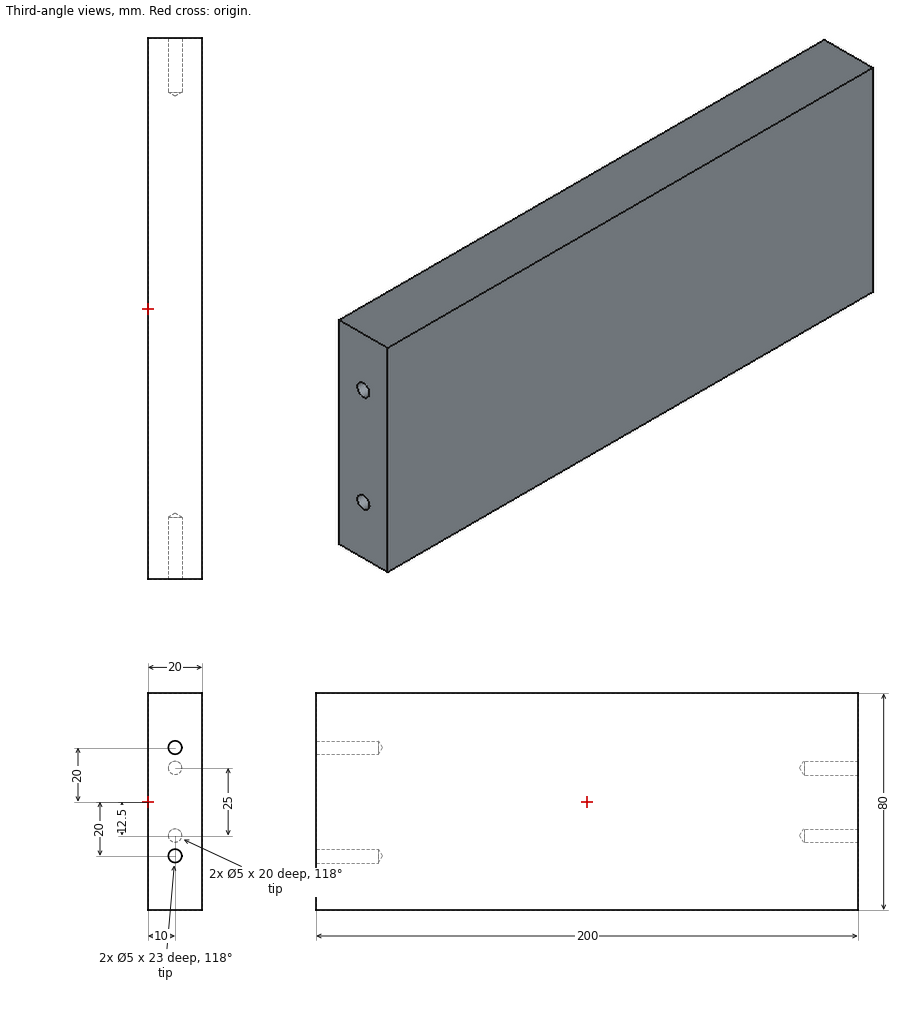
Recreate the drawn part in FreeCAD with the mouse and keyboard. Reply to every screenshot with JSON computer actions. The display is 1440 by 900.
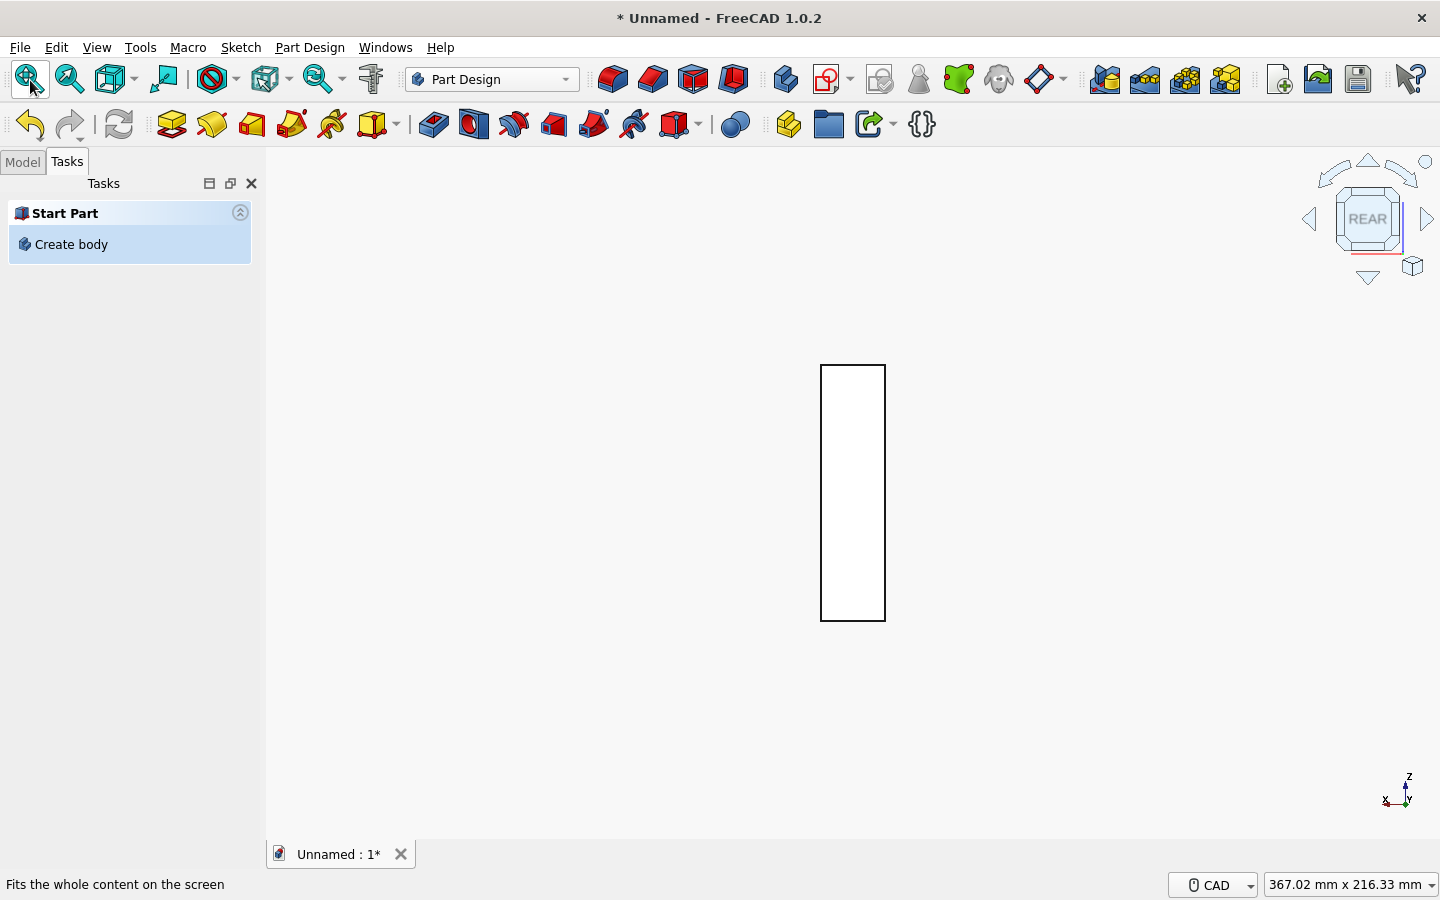
{"action": "left_click", "coordinate": [30, 80]}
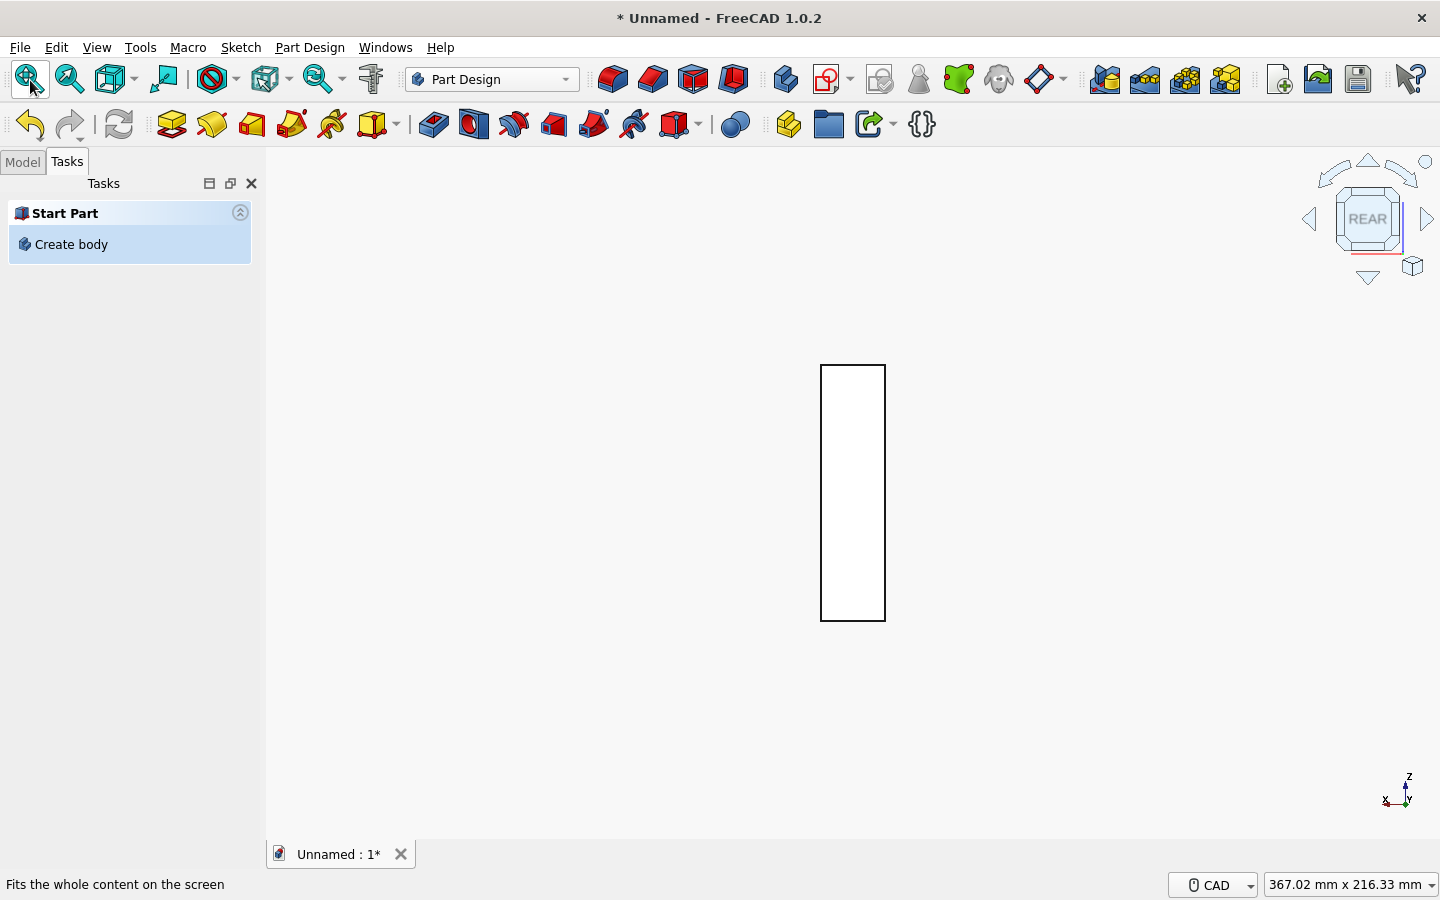
{"action": "left_click", "coordinate": [853, 565]}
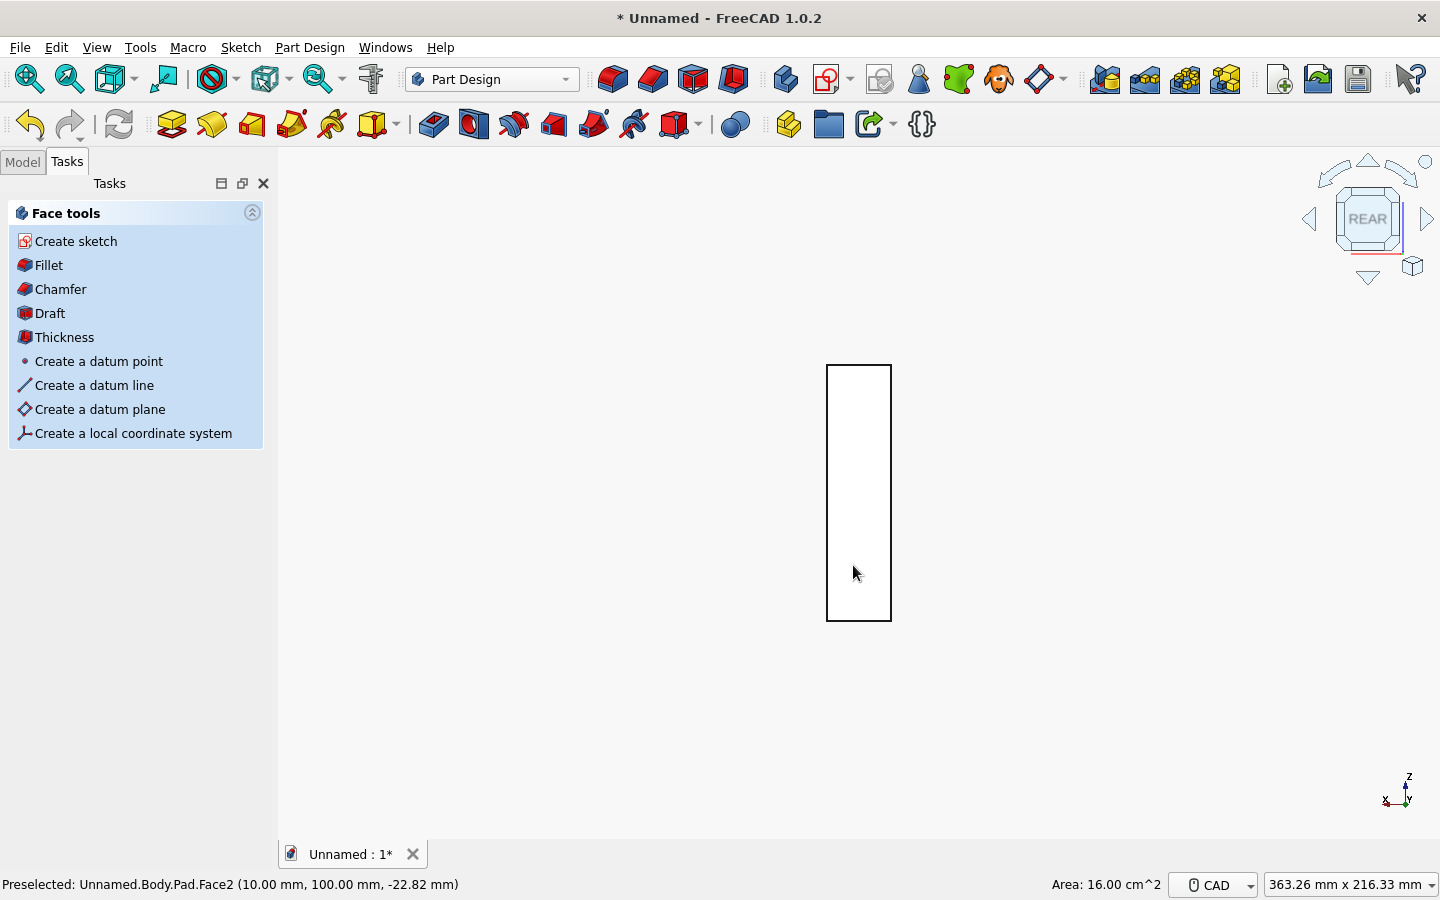
{"action": "left_click", "coordinate": [826, 80]}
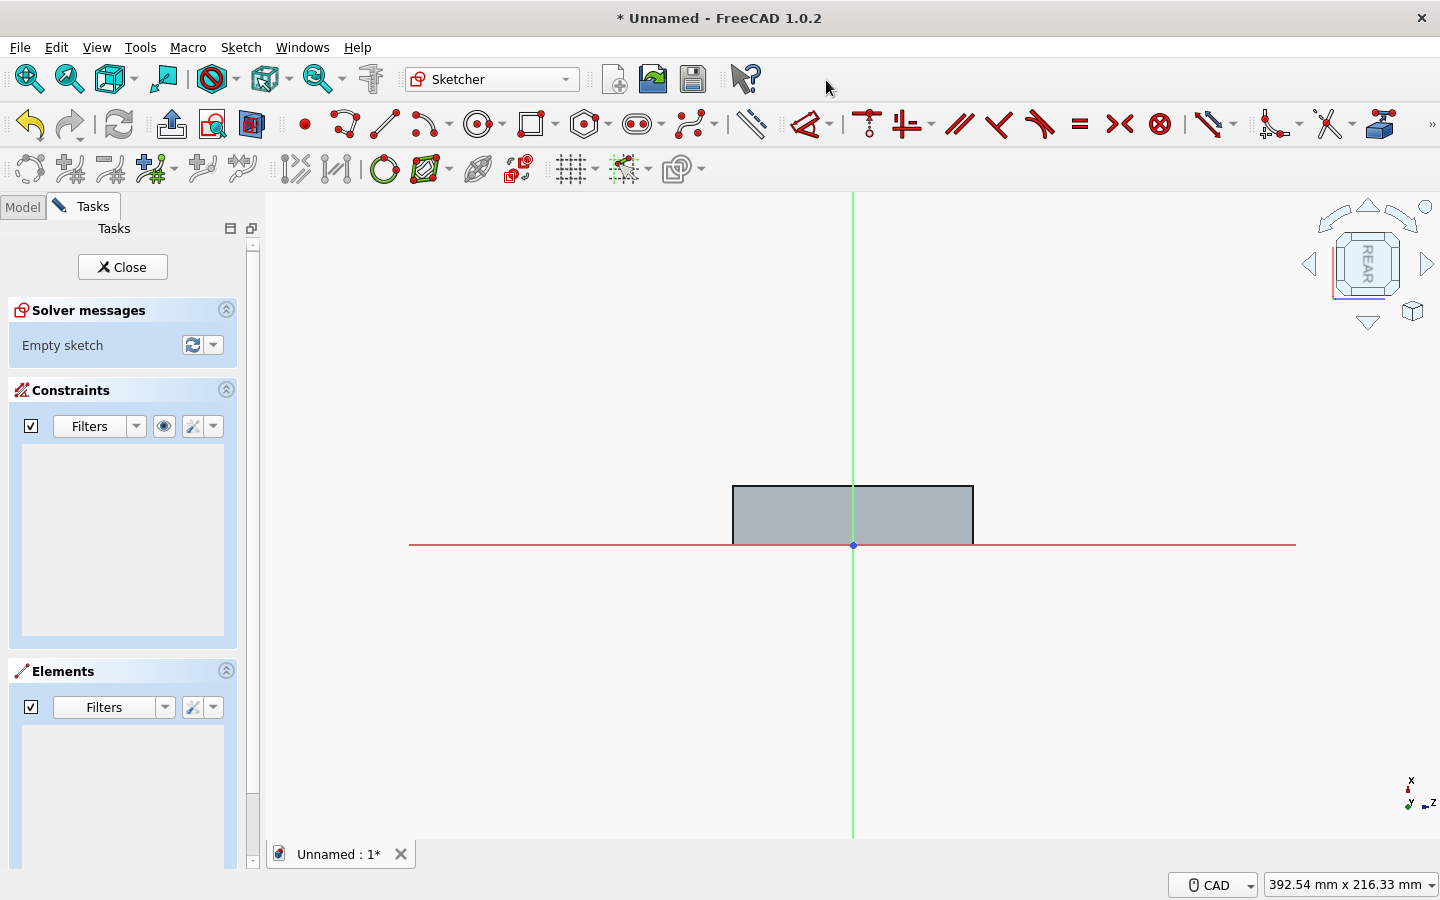
{"action": "scroll", "coordinate": [864, 528], "scroll_direction": "up", "scroll_amount": 10}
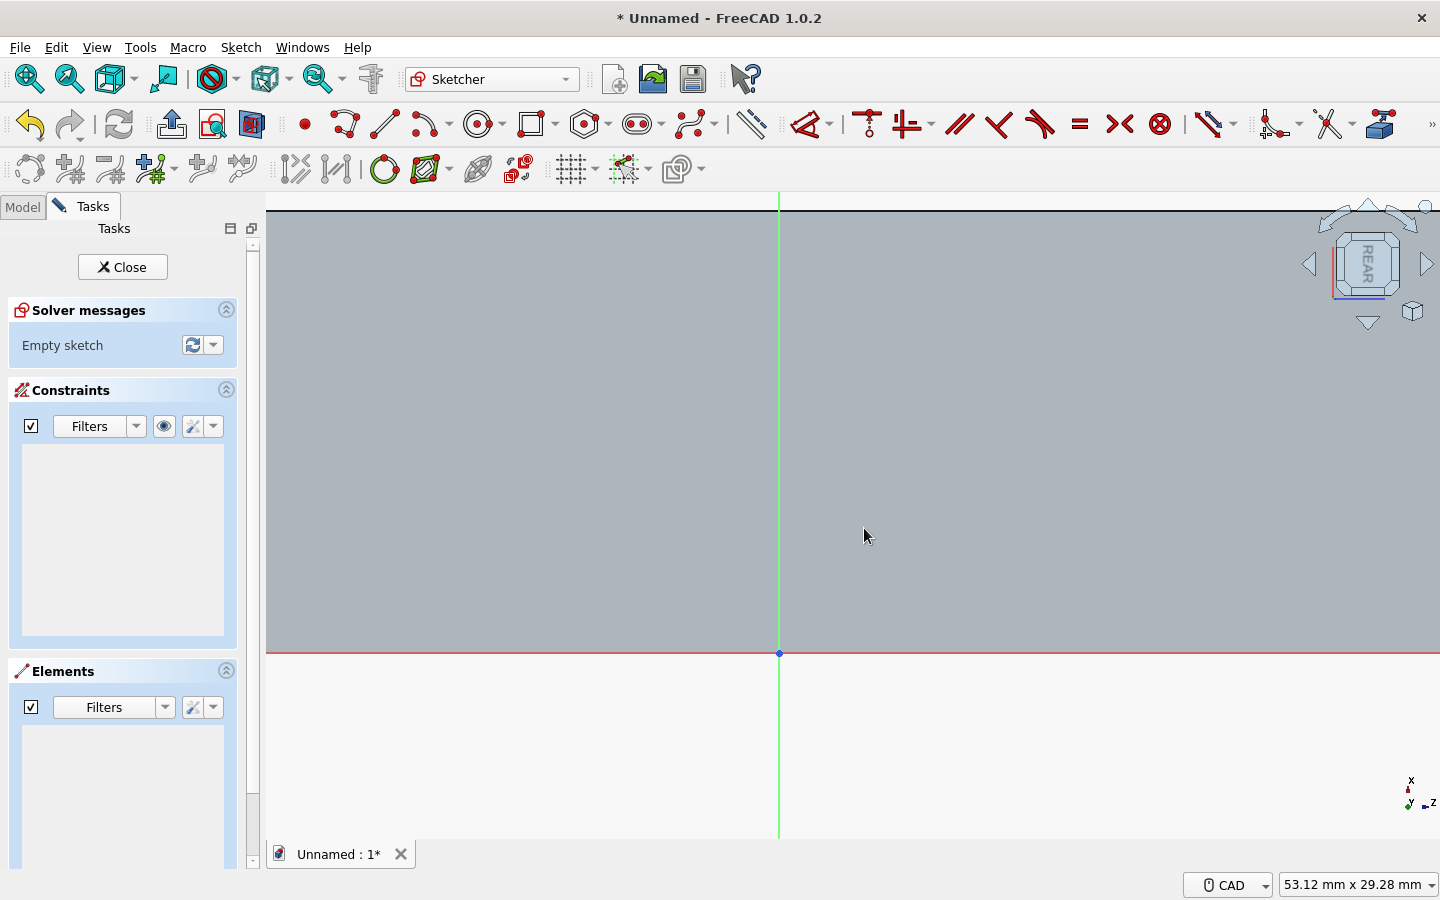
{"action": "left_click", "coordinate": [478, 124]}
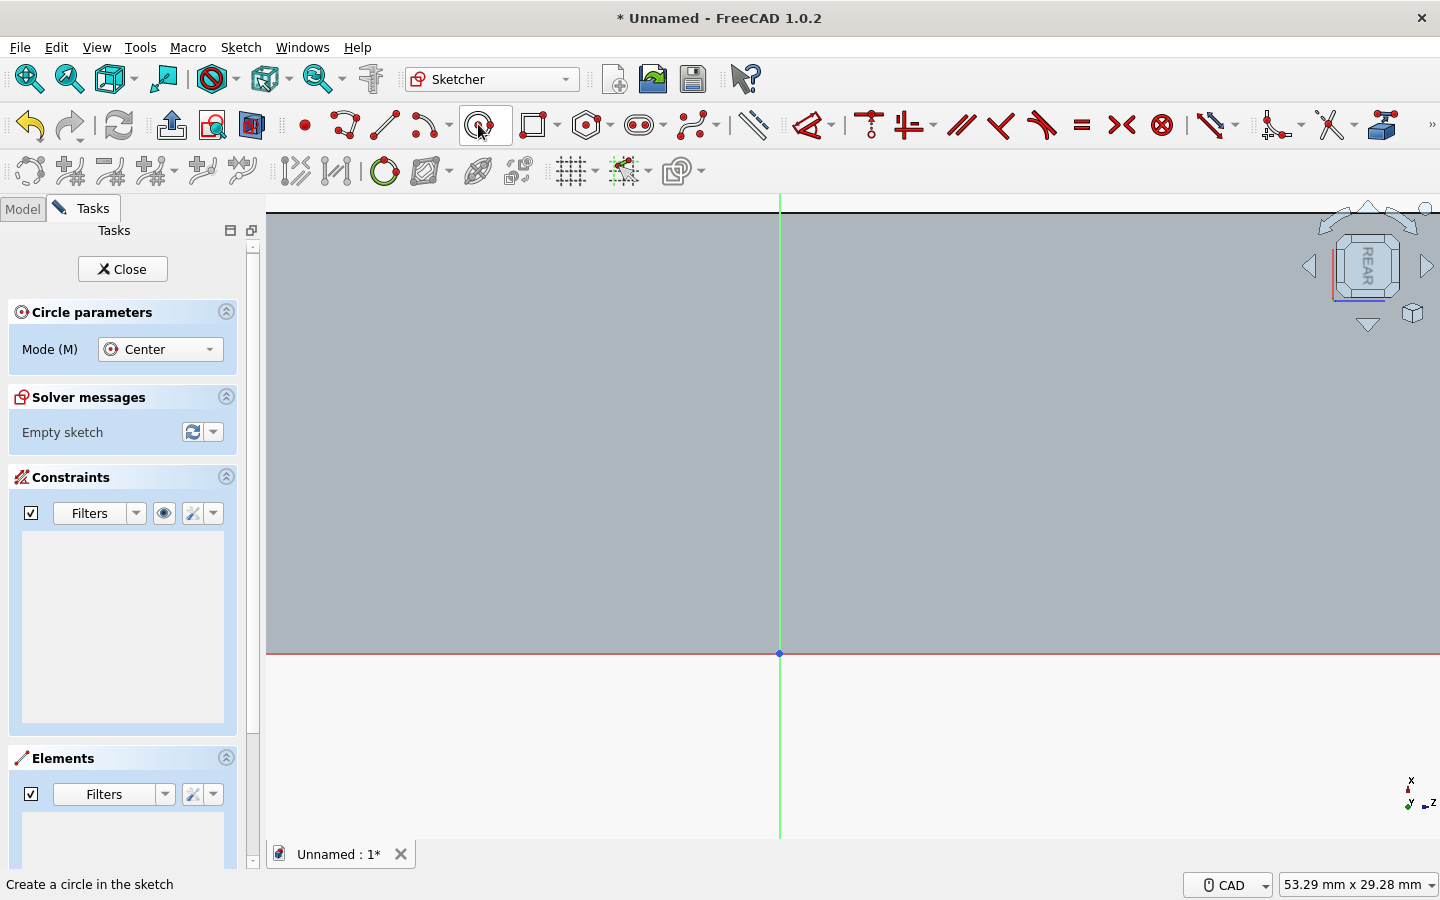
{"action": "left_click", "coordinate": [504, 434]}
{"action": "mouse_move", "coordinate": [543, 395]}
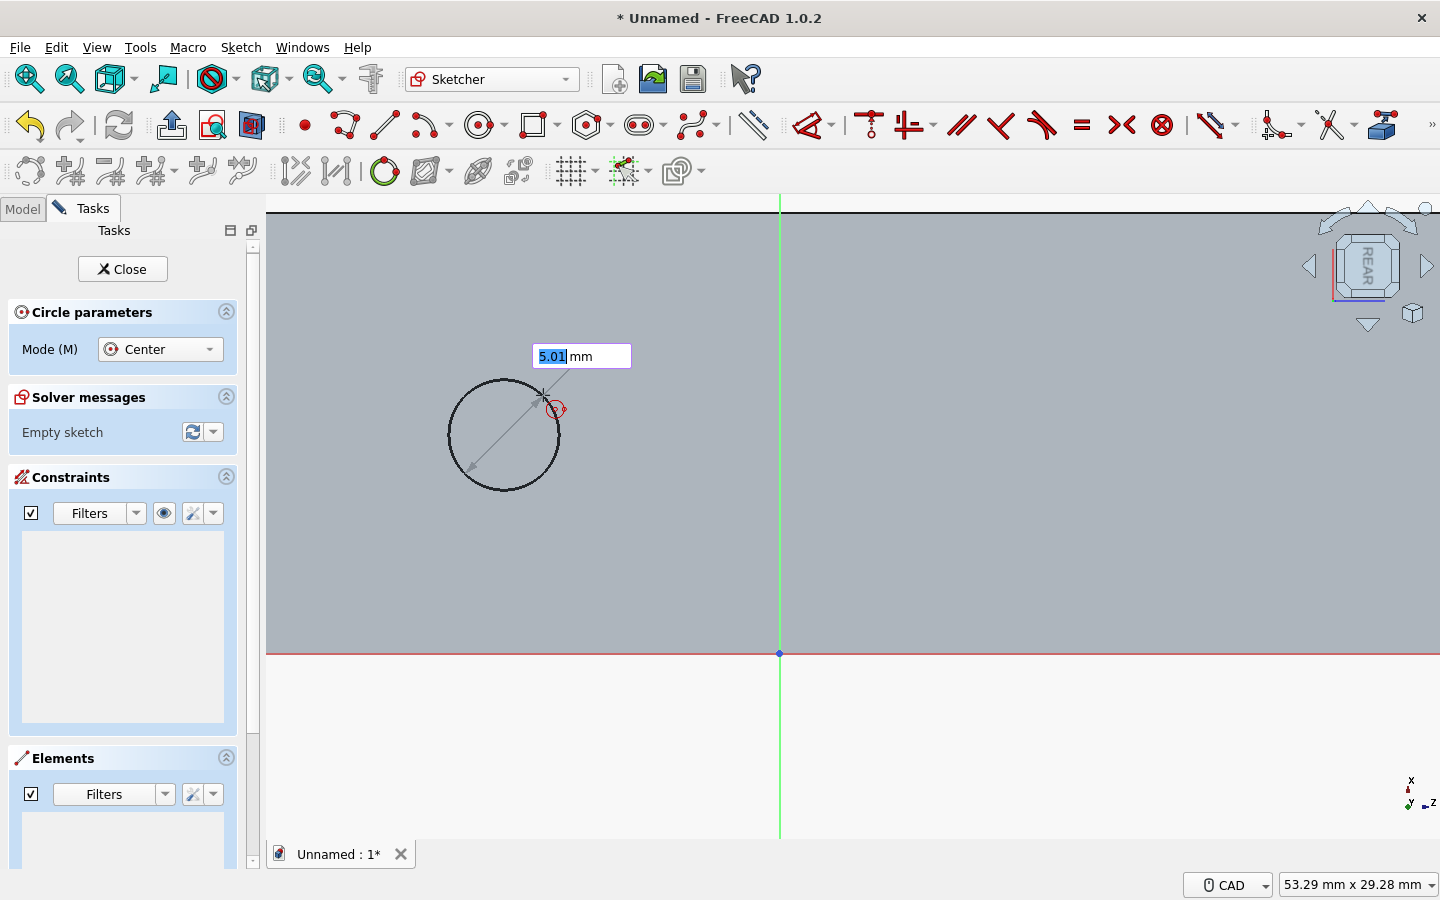
{"action": "type", "text": "5"}
{"action": "key", "text": "Return"}